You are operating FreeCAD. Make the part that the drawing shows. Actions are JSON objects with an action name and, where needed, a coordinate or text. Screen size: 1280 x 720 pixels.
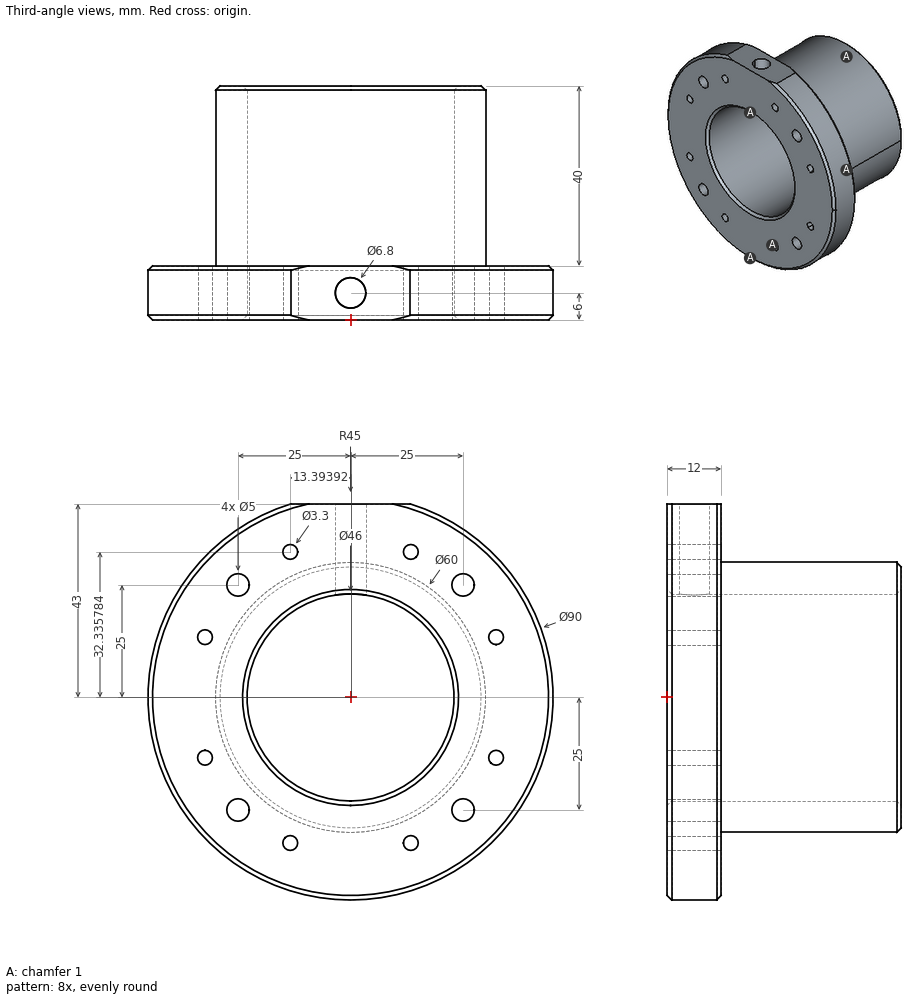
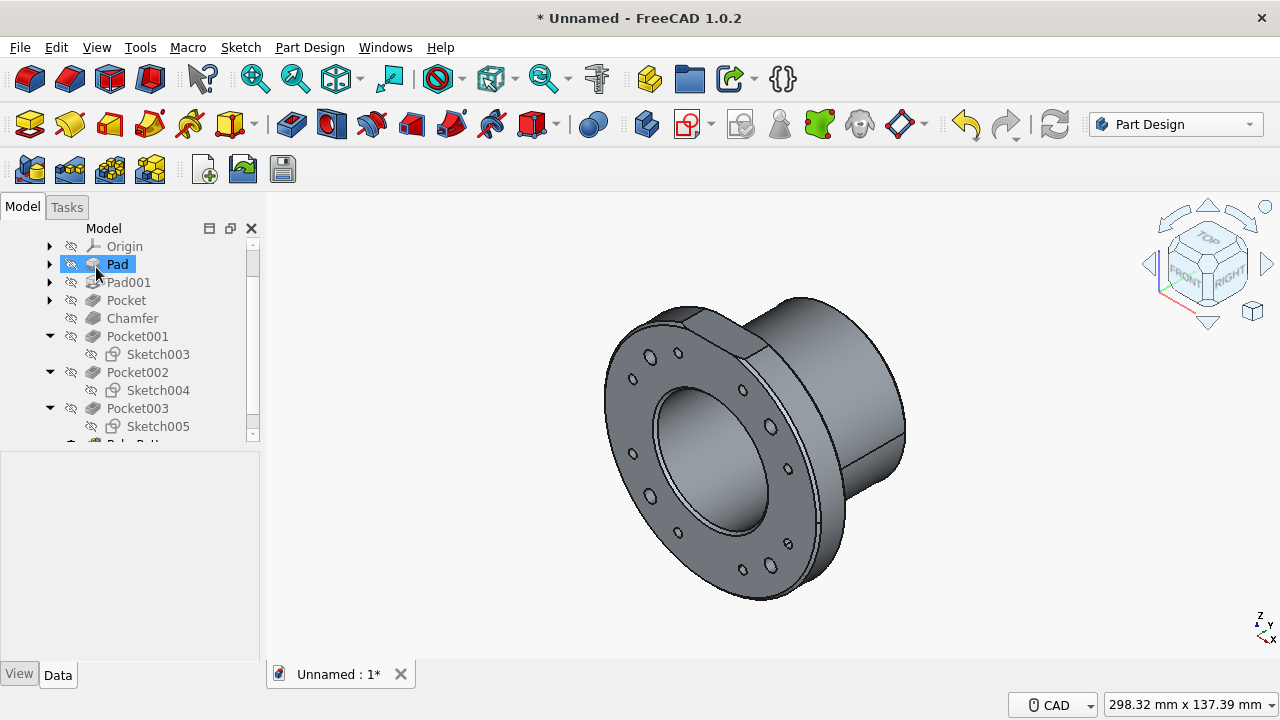
{"action": "left_click", "coordinate": [734, 338]}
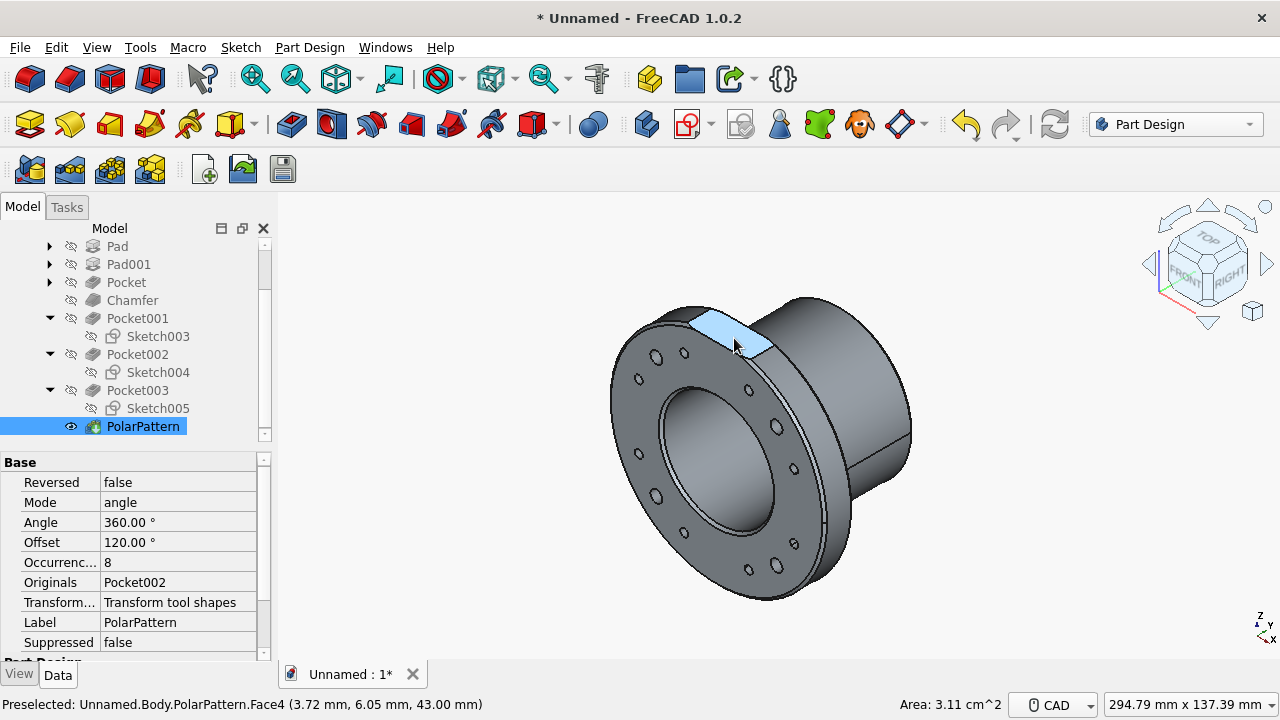
{"action": "left_click", "coordinate": [688, 124]}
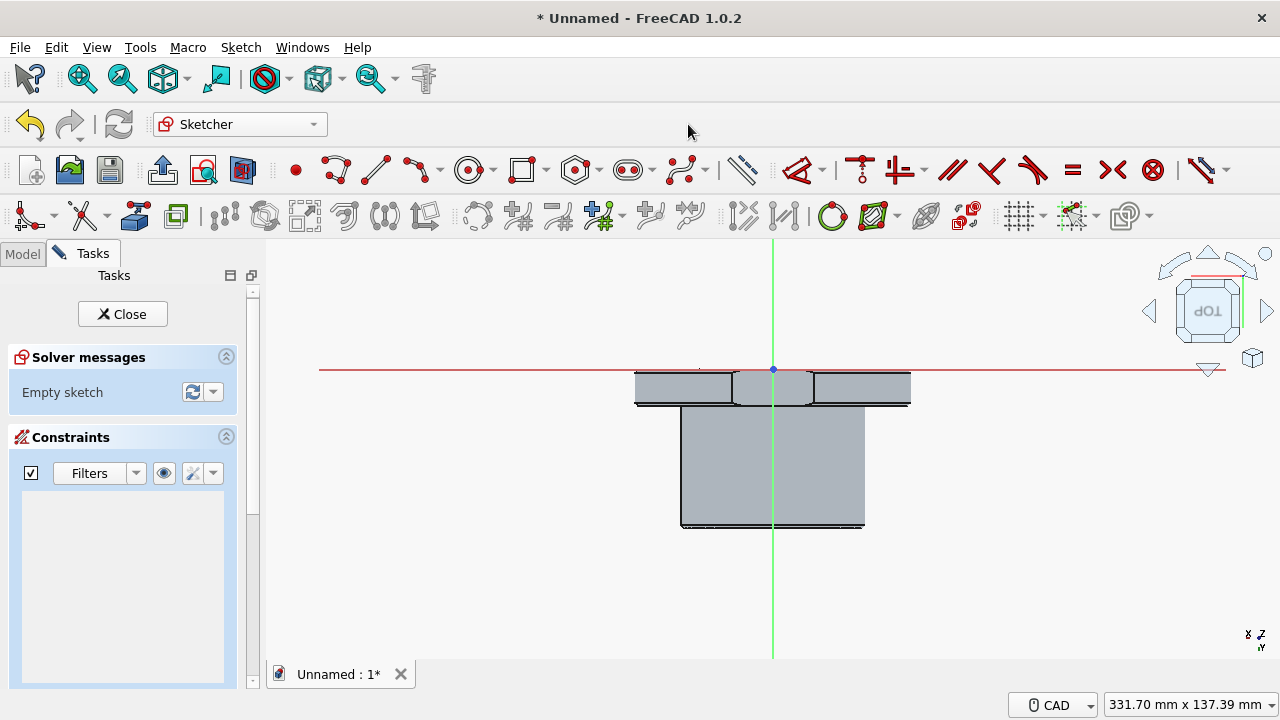
{"action": "scroll", "coordinate": [782, 376], "scroll_direction": "up", "scroll_amount": 11}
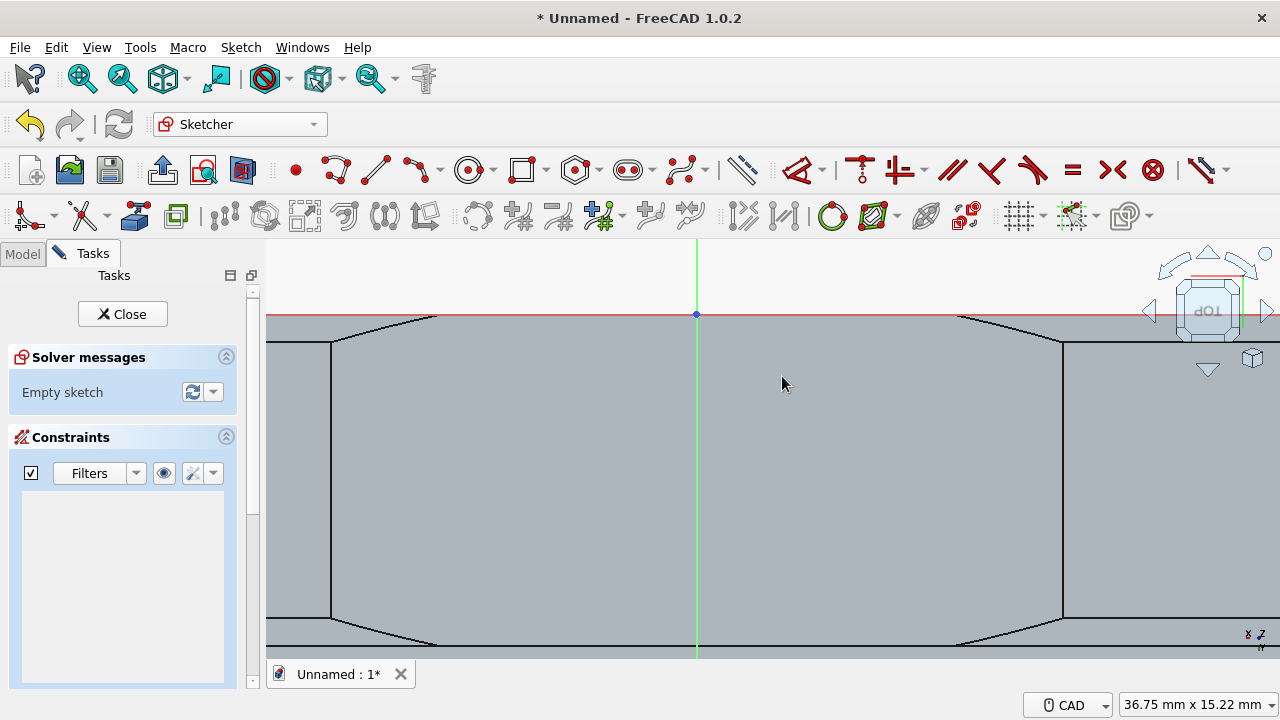
{"action": "left_click", "coordinate": [470, 170]}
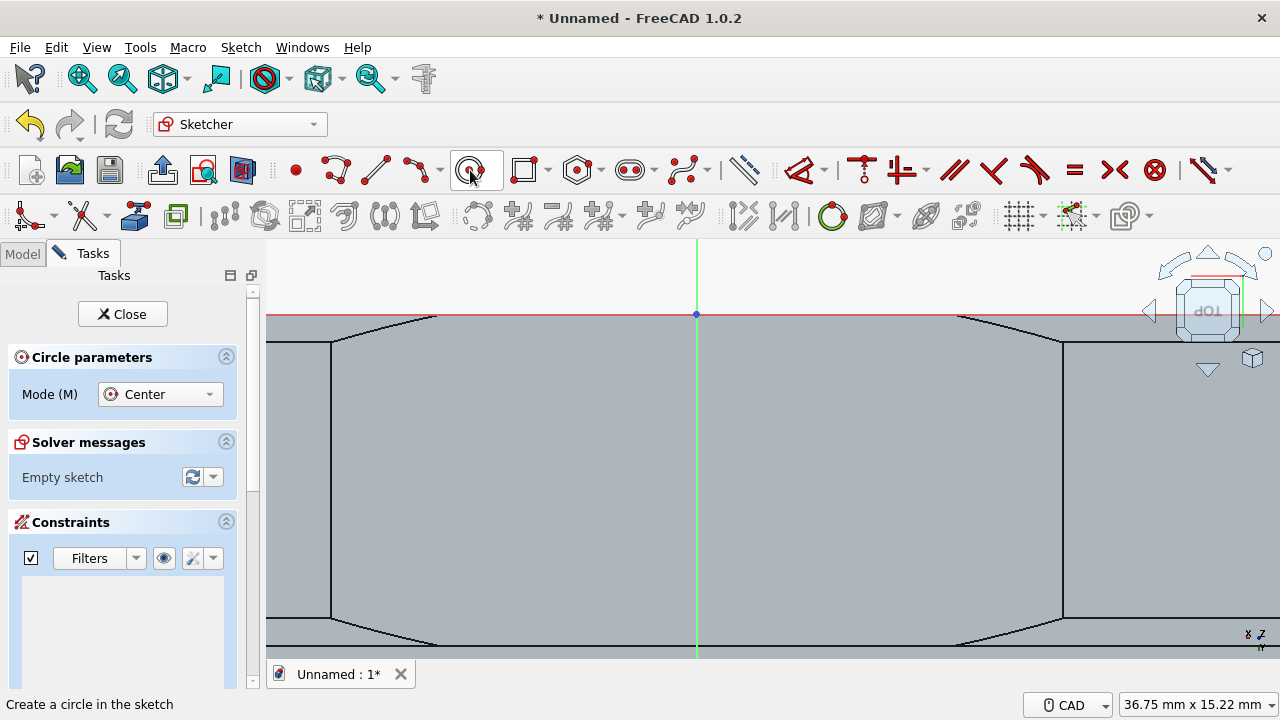
{"action": "left_click", "coordinate": [697, 480]}
{"action": "left_click", "coordinate": [763, 414]}
{"action": "key", "text": "Escape"}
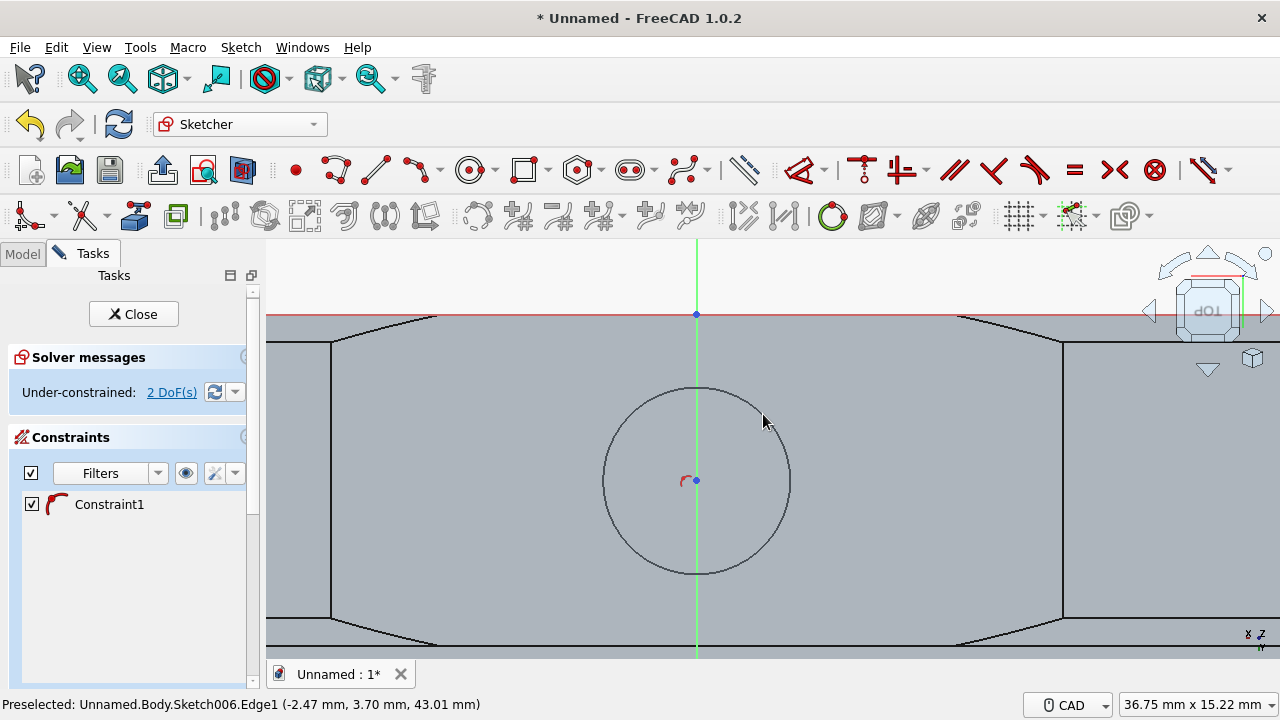
{"action": "left_click", "coordinate": [800, 170]}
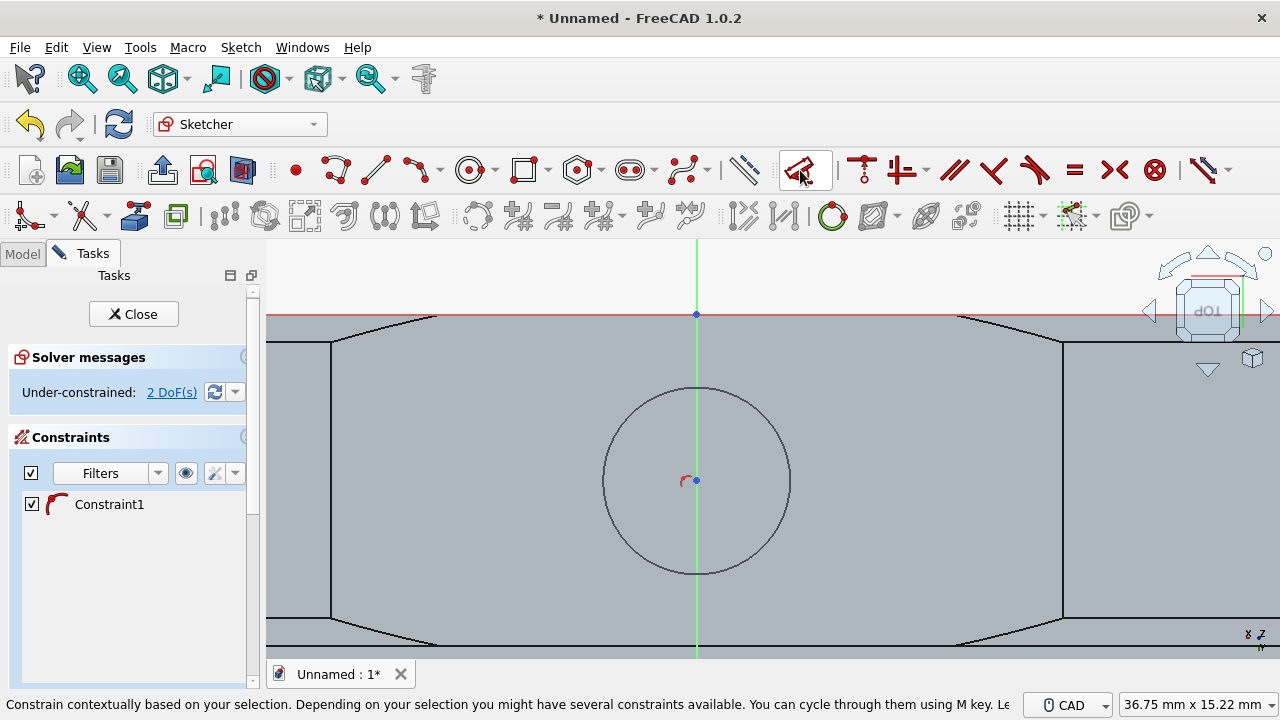
{"action": "left_click", "coordinate": [763, 415]}
{"action": "left_click", "coordinate": [786, 392]}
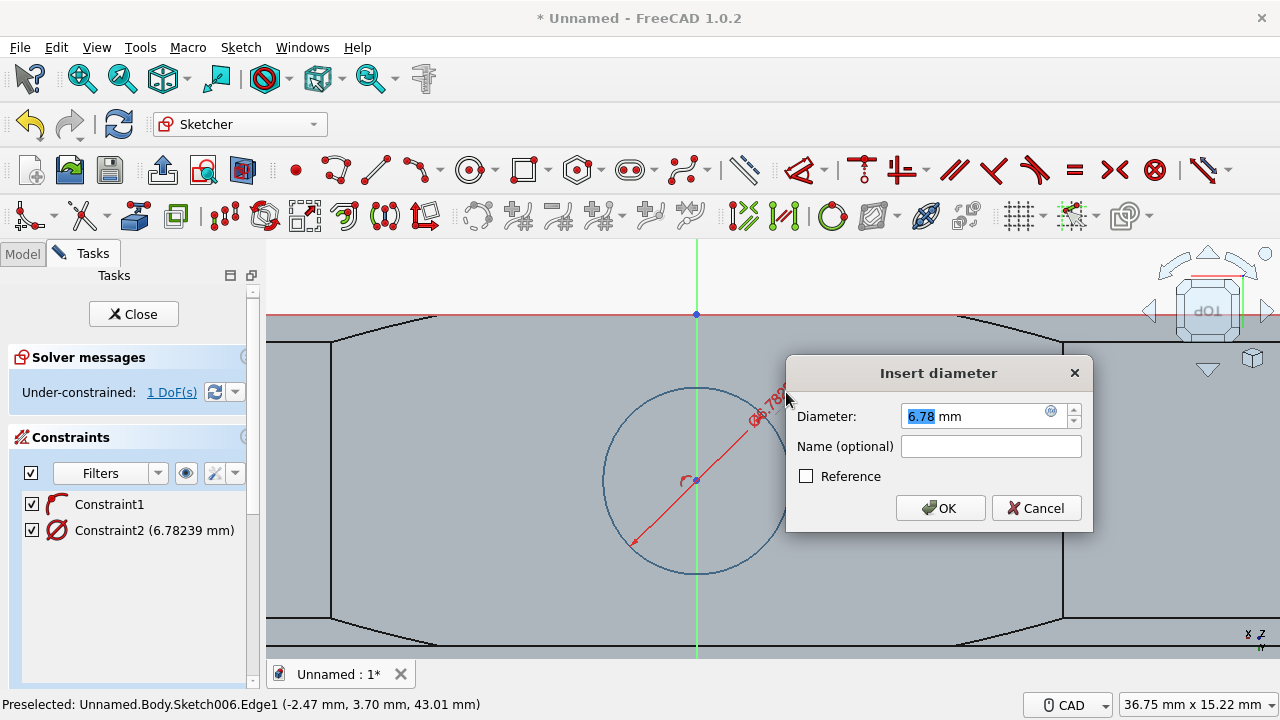
{"action": "type", "text": "6.8"}
{"action": "key", "text": "Return"}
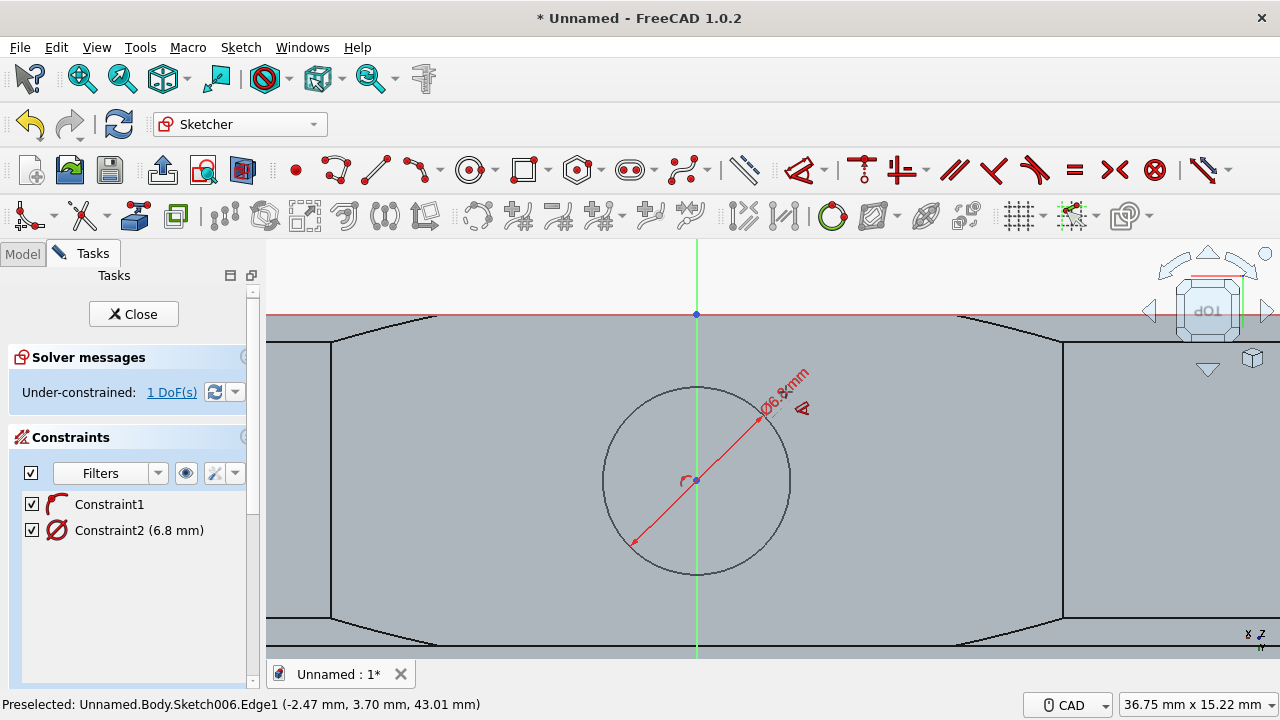
{"action": "left_click", "coordinate": [697, 481]}
{"action": "left_click", "coordinate": [731, 360]}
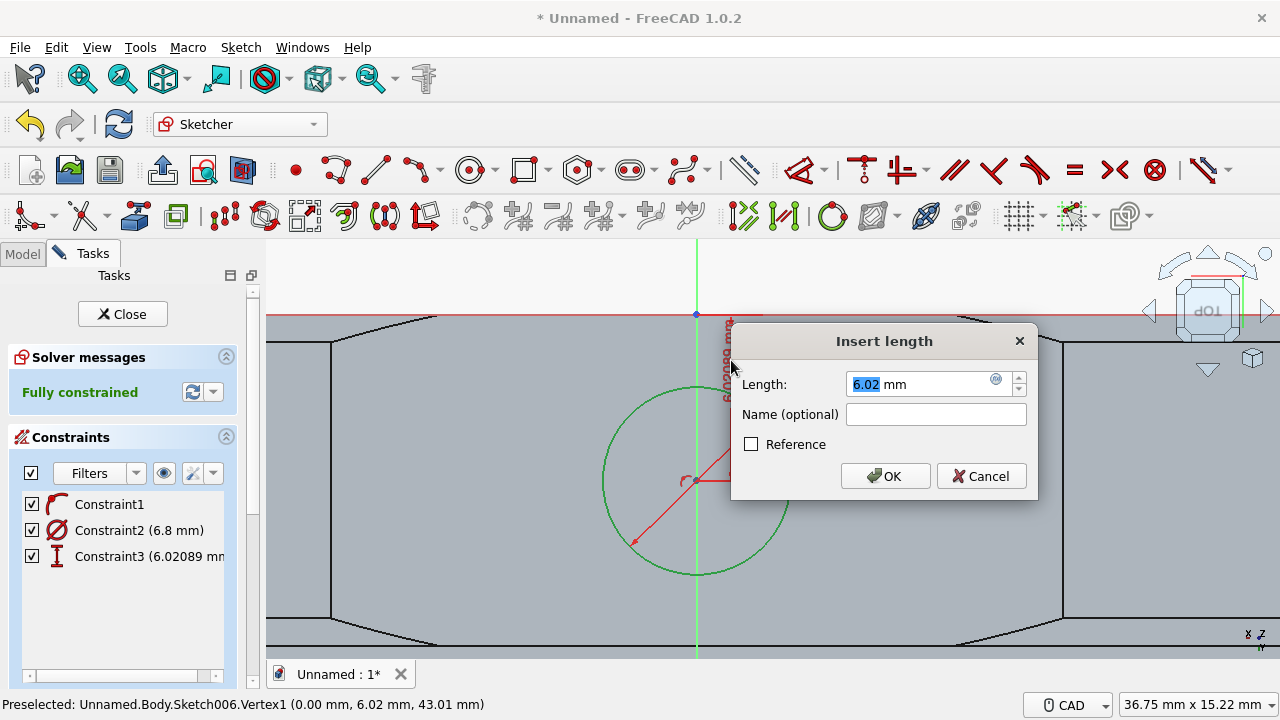
{"action": "type", "text": "6"}
{"action": "key", "text": "Return"}
{"action": "key", "text": "Escape"}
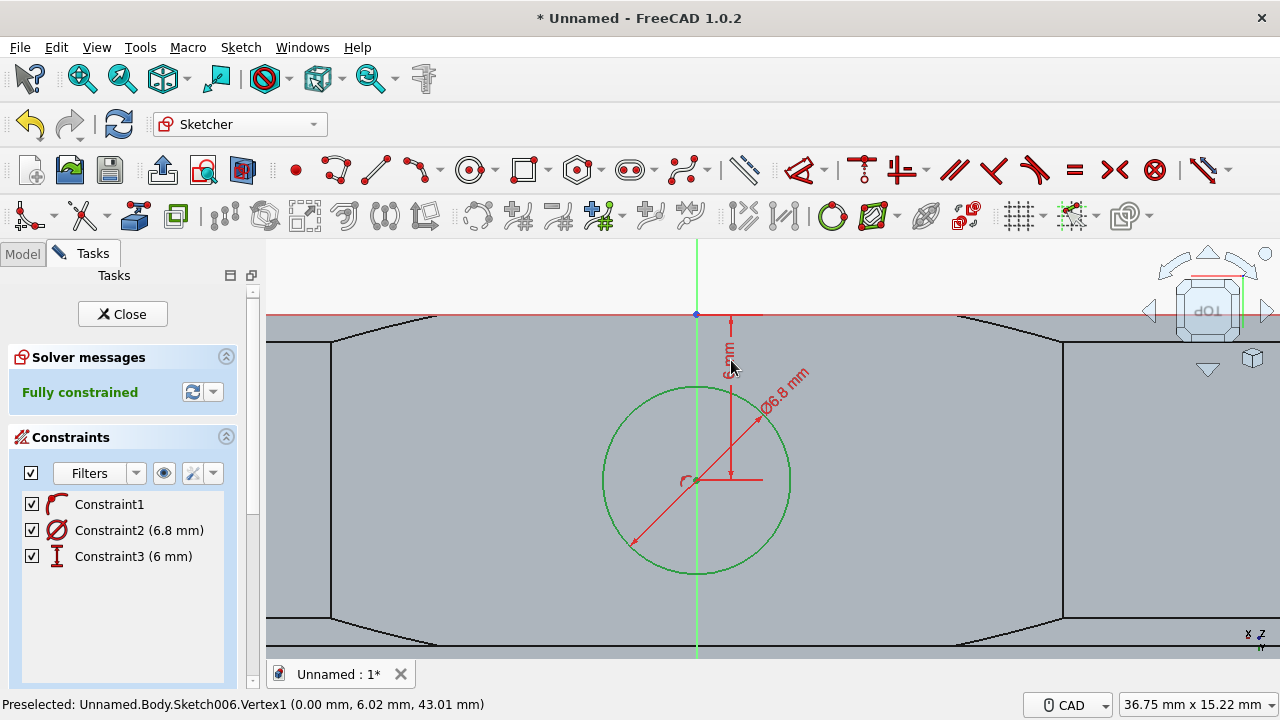
{"action": "left_click", "coordinate": [123, 314]}